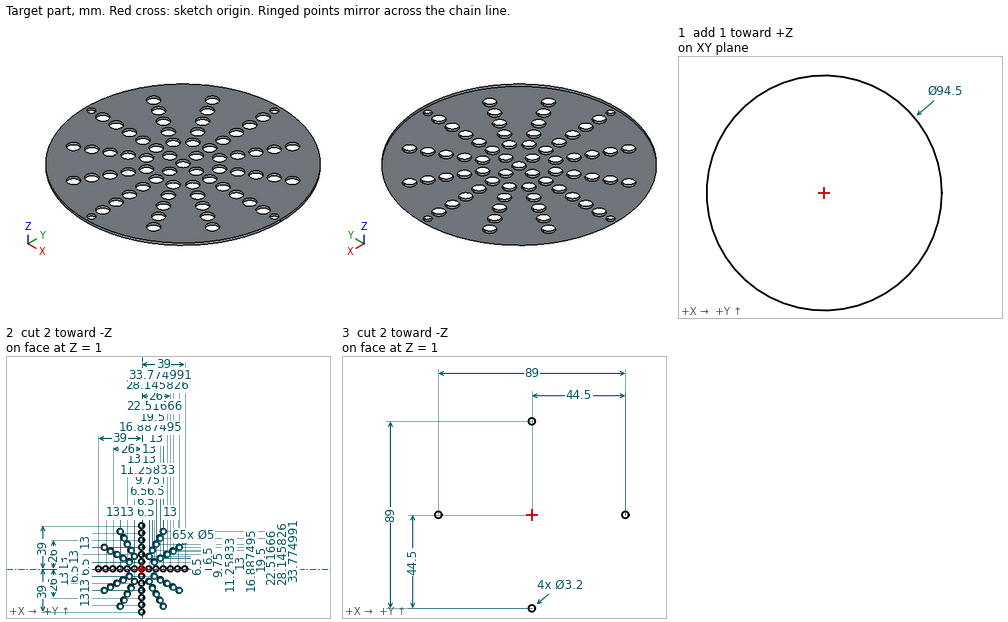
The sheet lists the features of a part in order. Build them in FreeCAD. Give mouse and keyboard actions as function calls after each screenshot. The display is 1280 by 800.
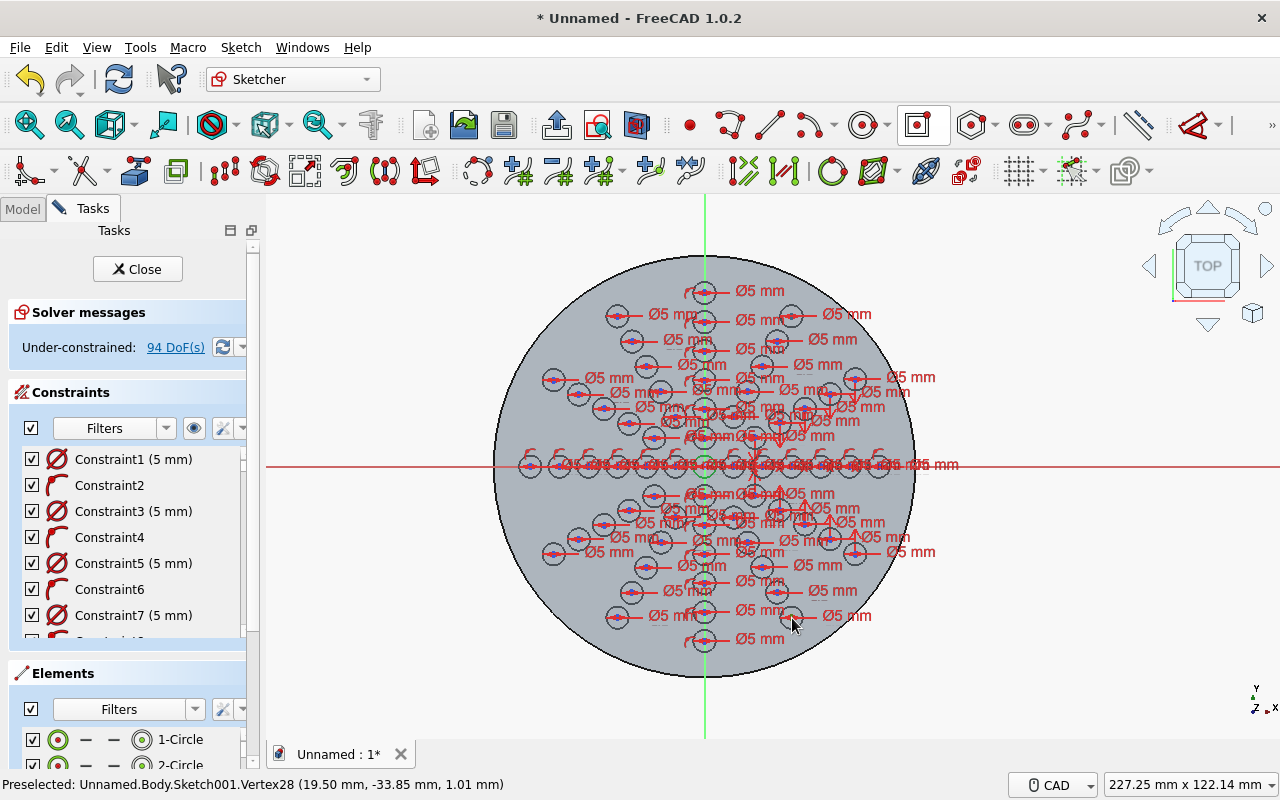
click(353, 467)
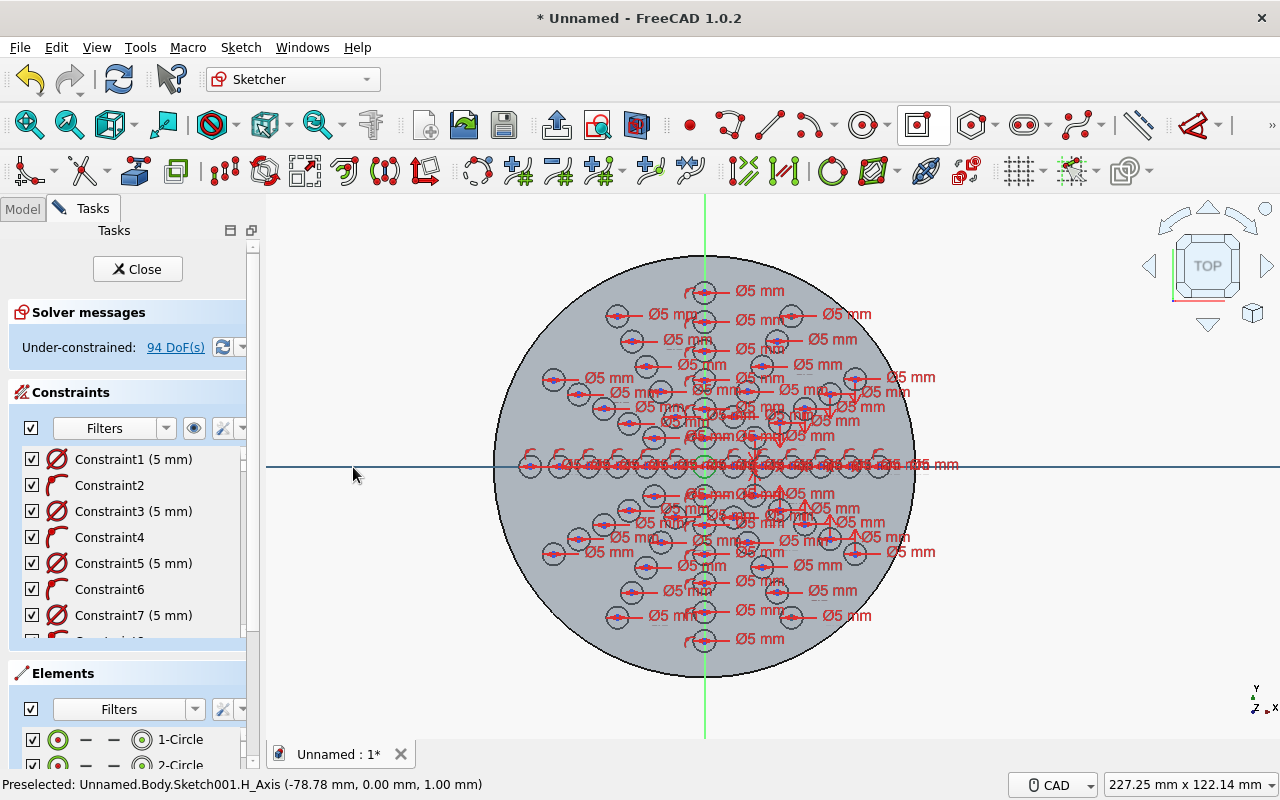
key(s)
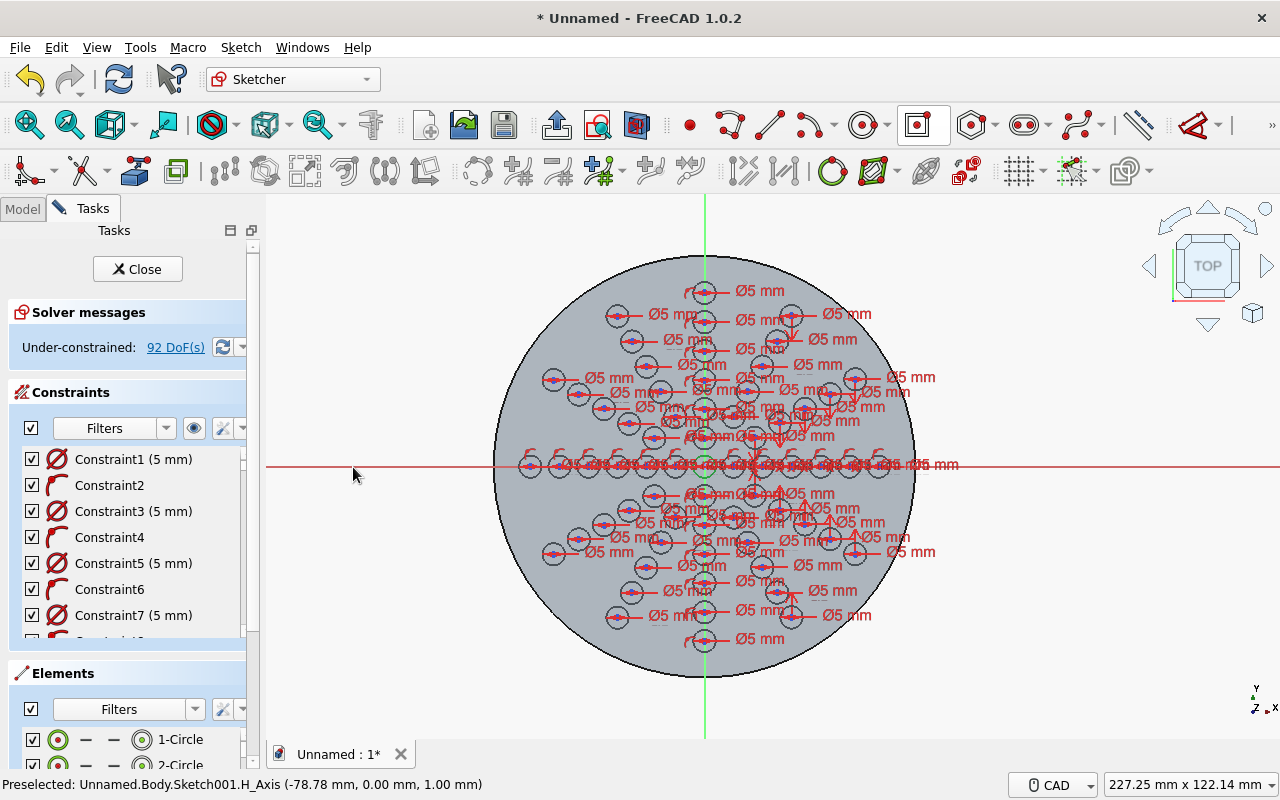
click(777, 341)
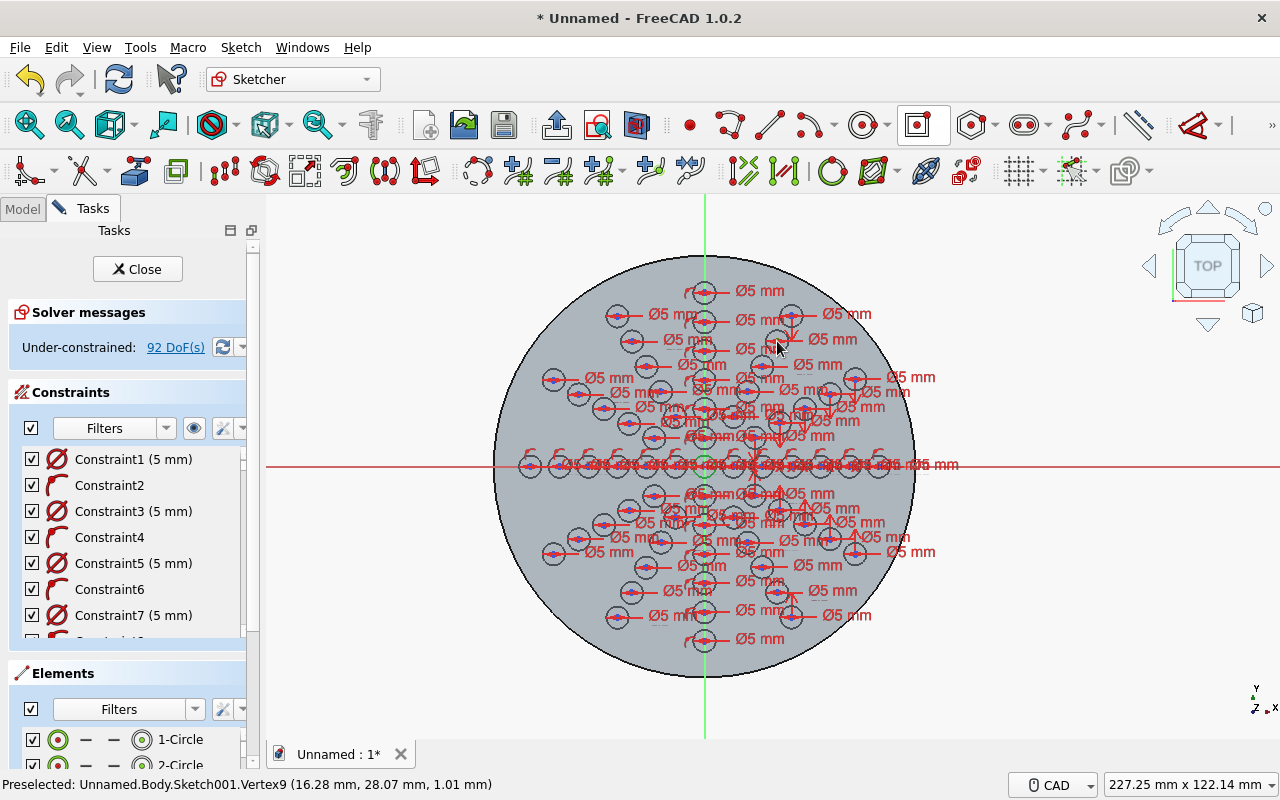
click(777, 593)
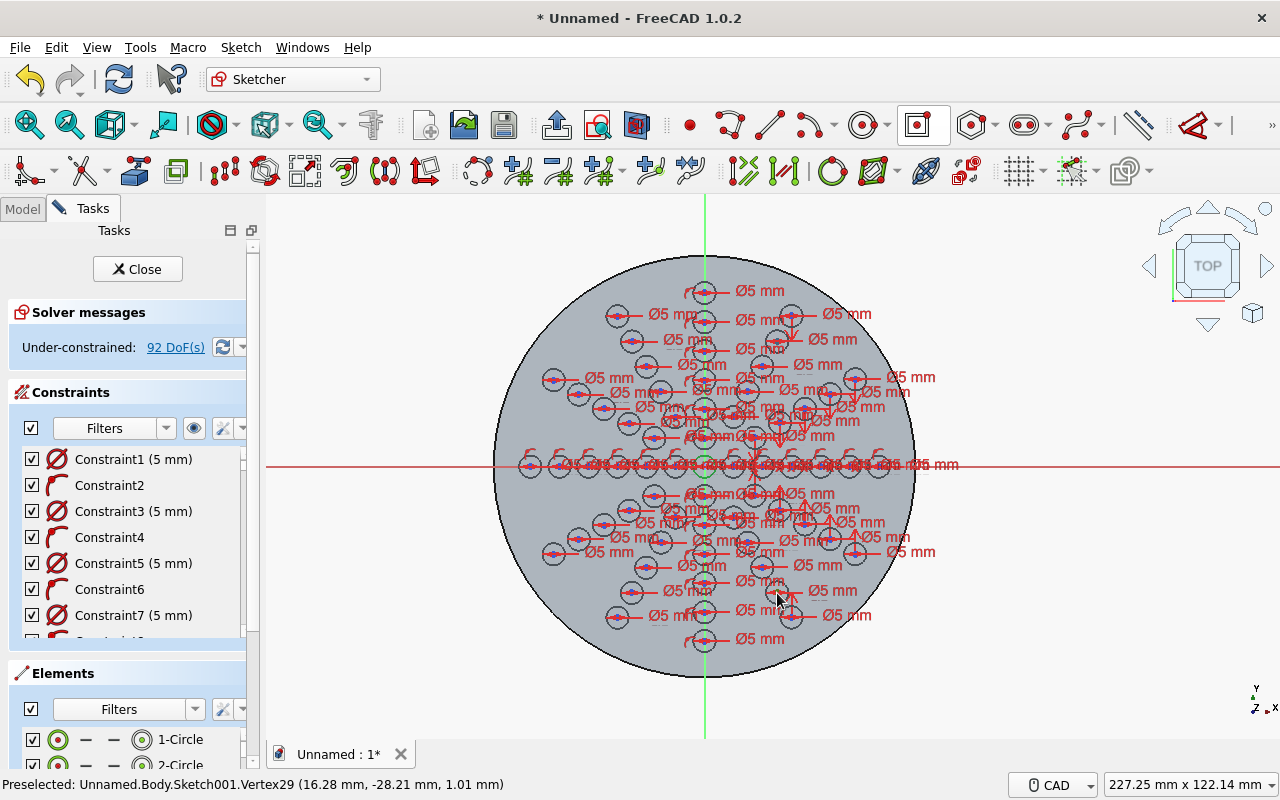
click(353, 467)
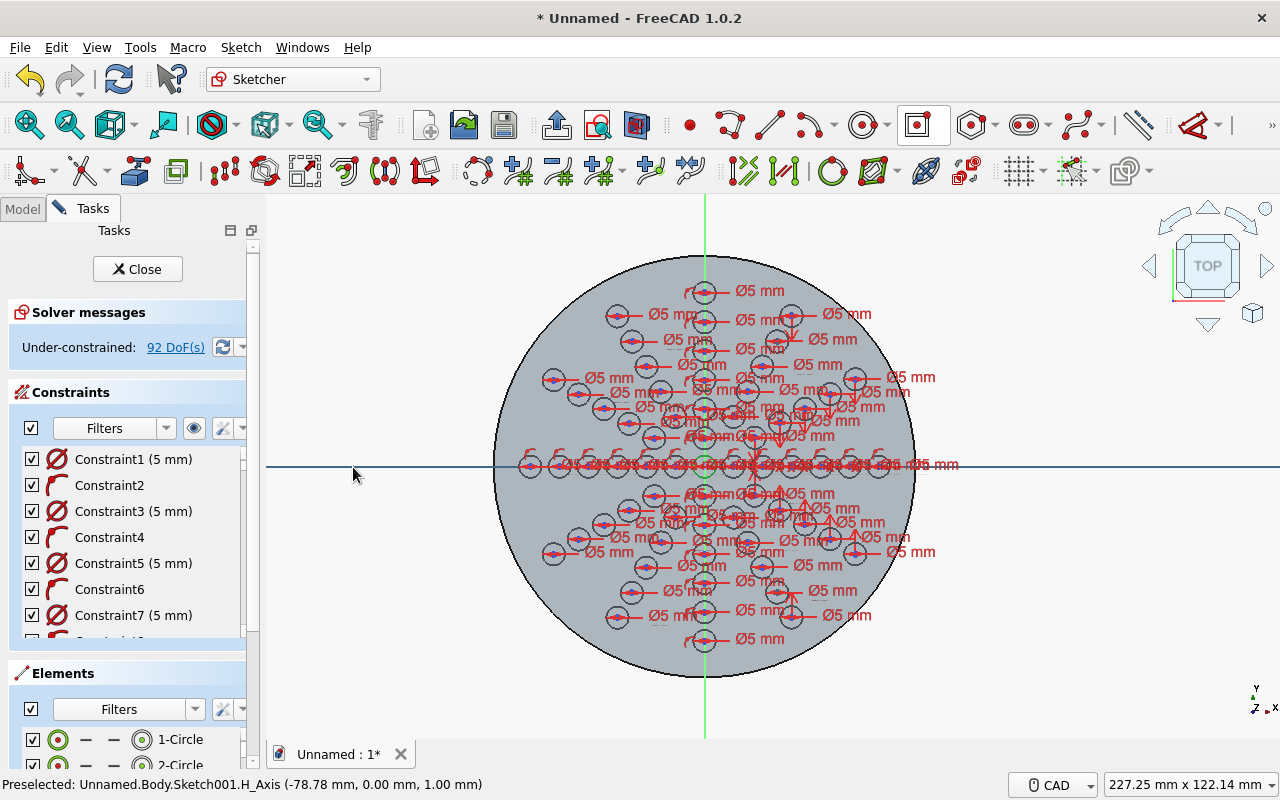
key(s)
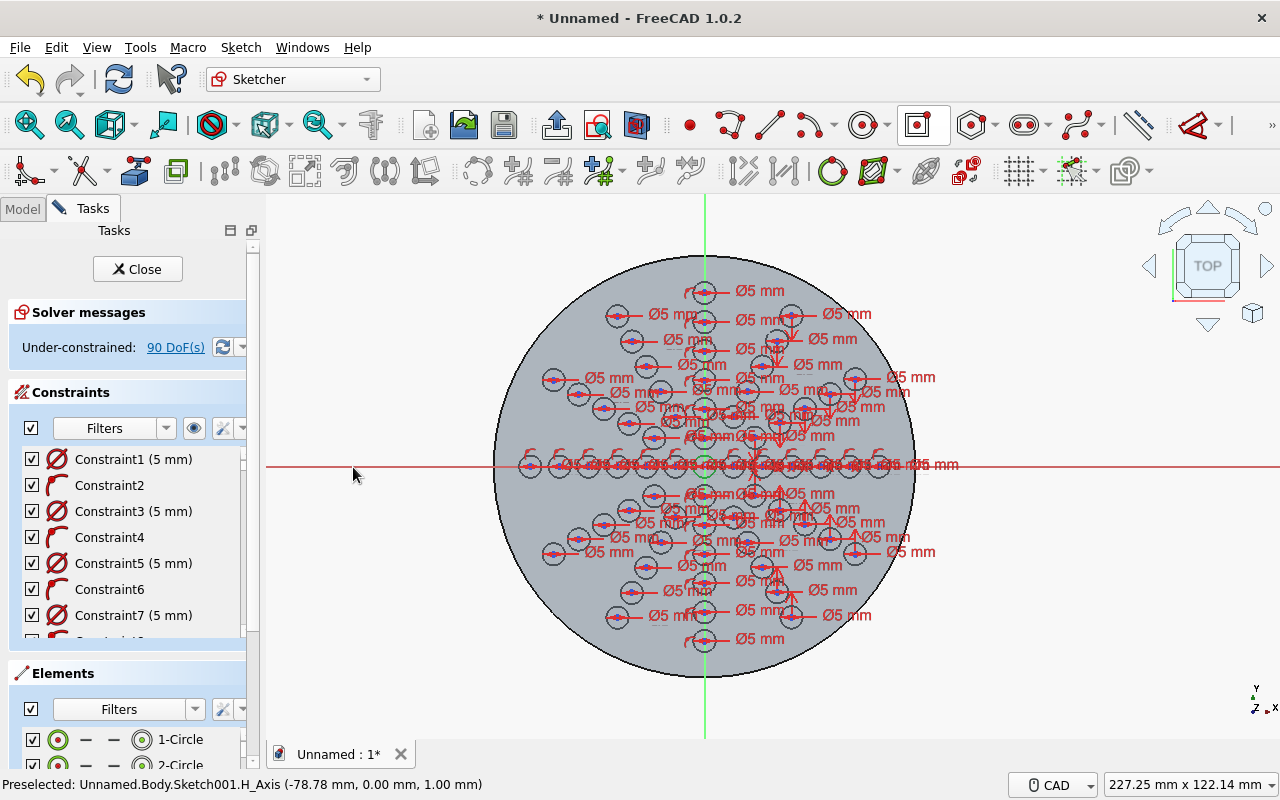
click(762, 367)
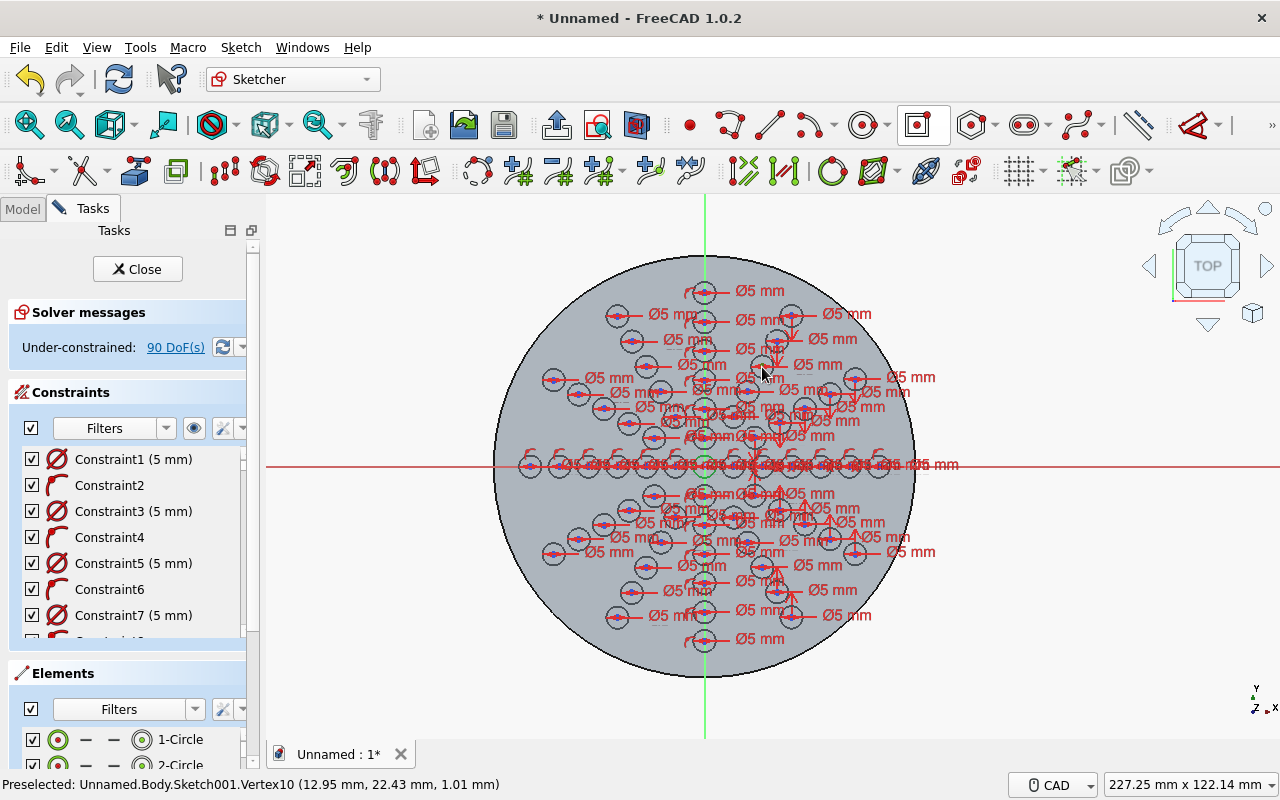
click(762, 567)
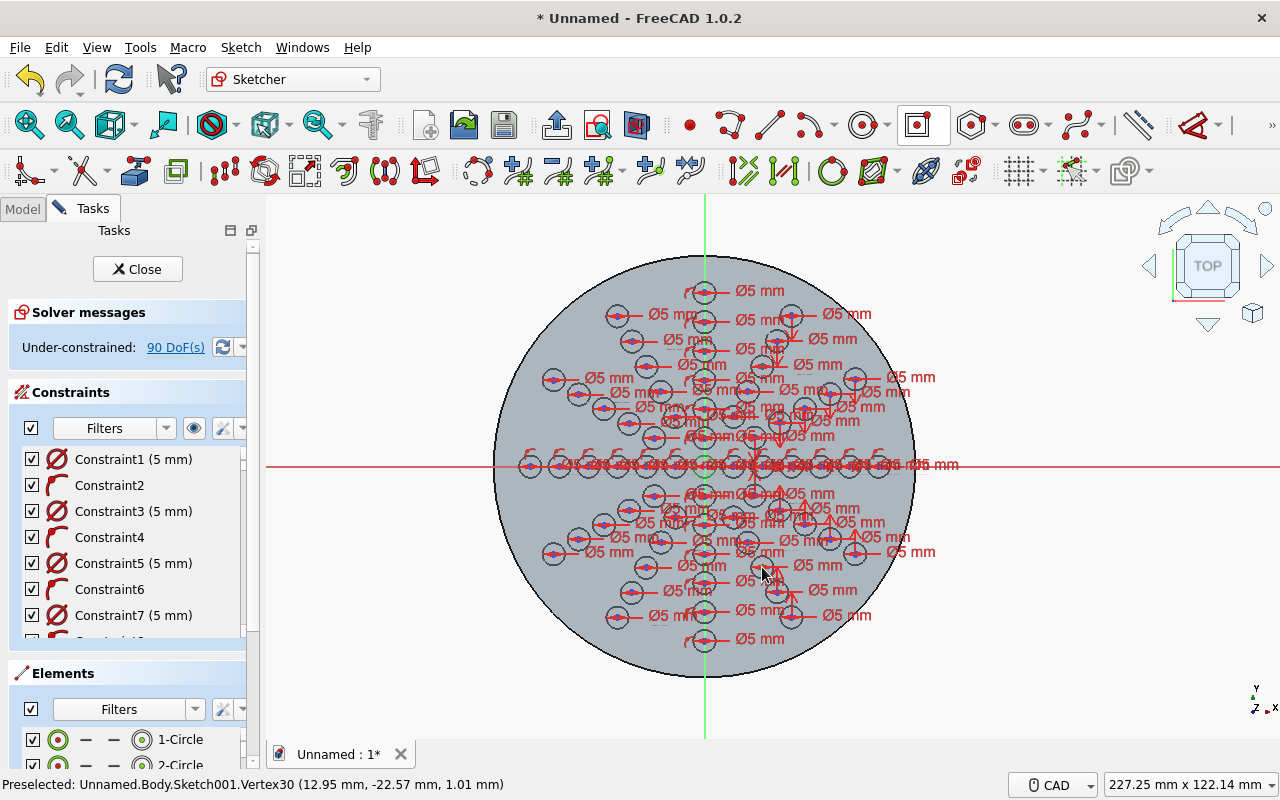
click(353, 467)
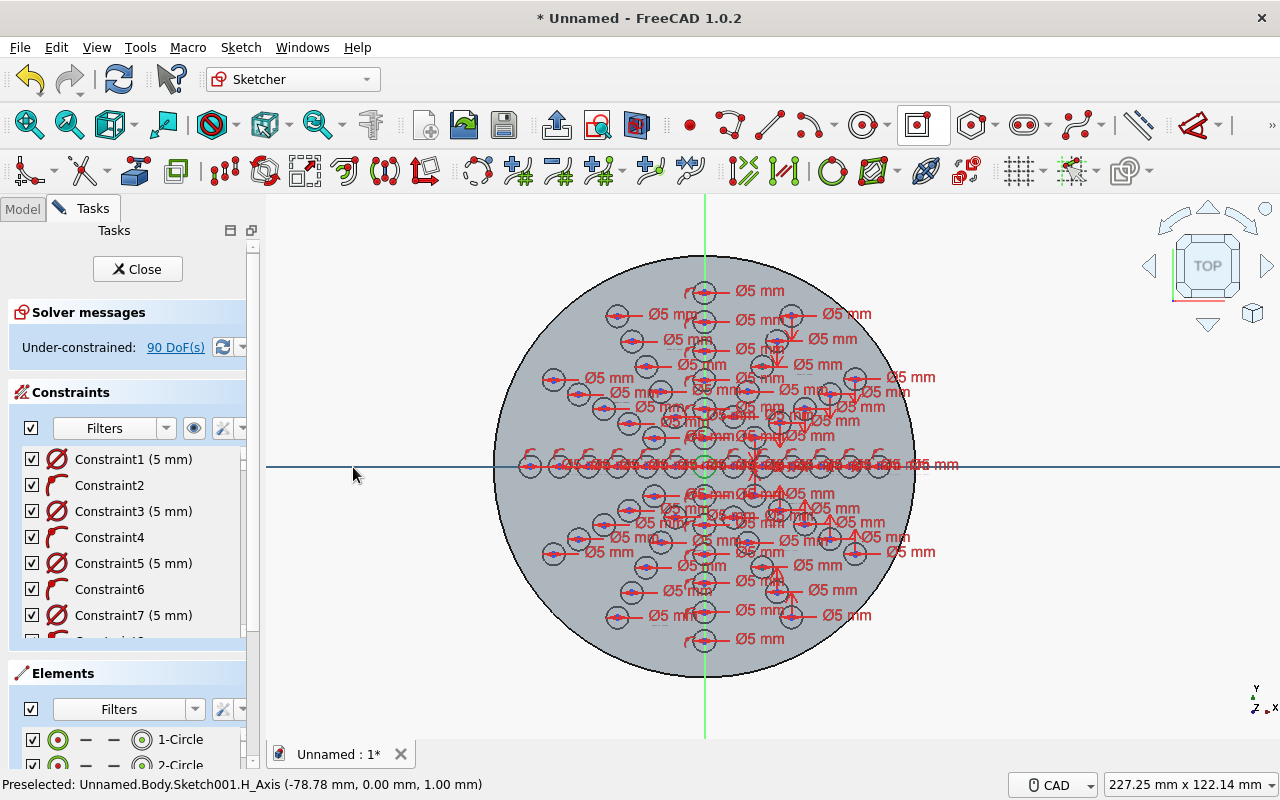
key(s)